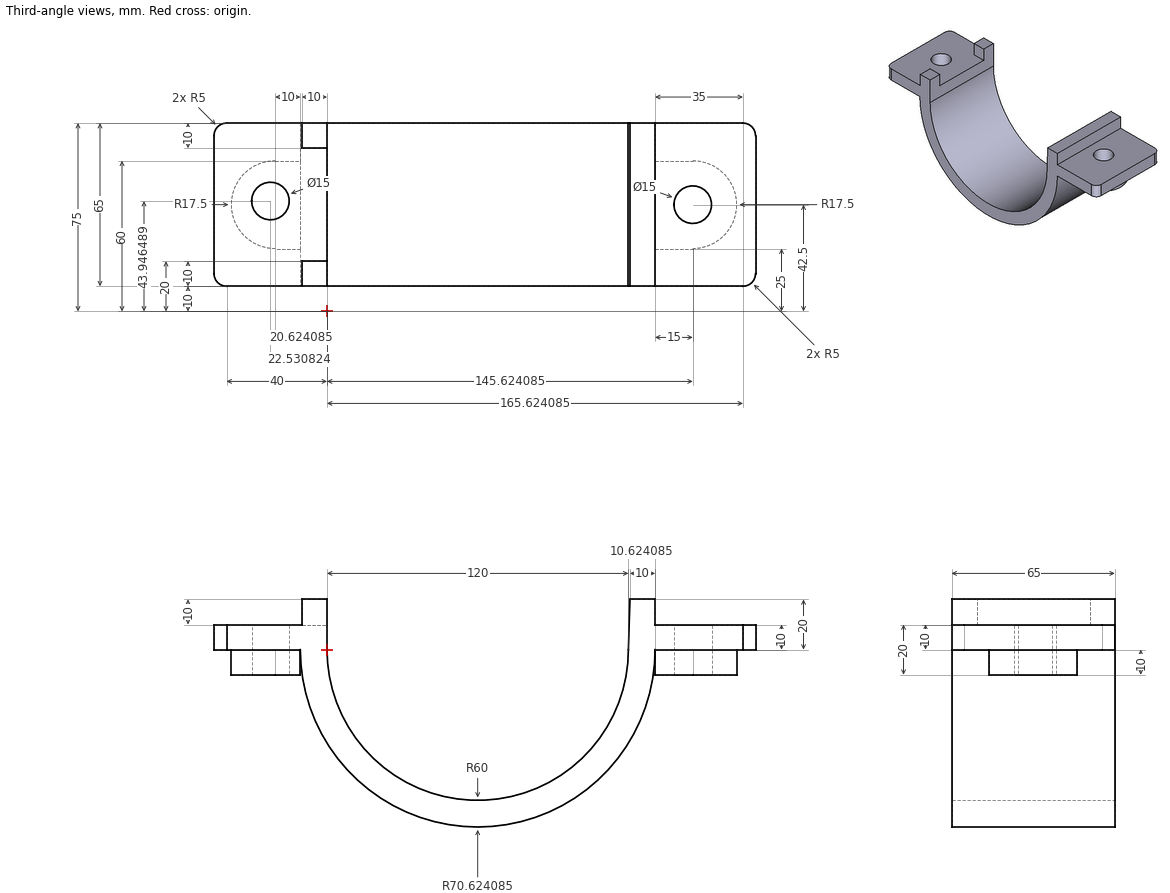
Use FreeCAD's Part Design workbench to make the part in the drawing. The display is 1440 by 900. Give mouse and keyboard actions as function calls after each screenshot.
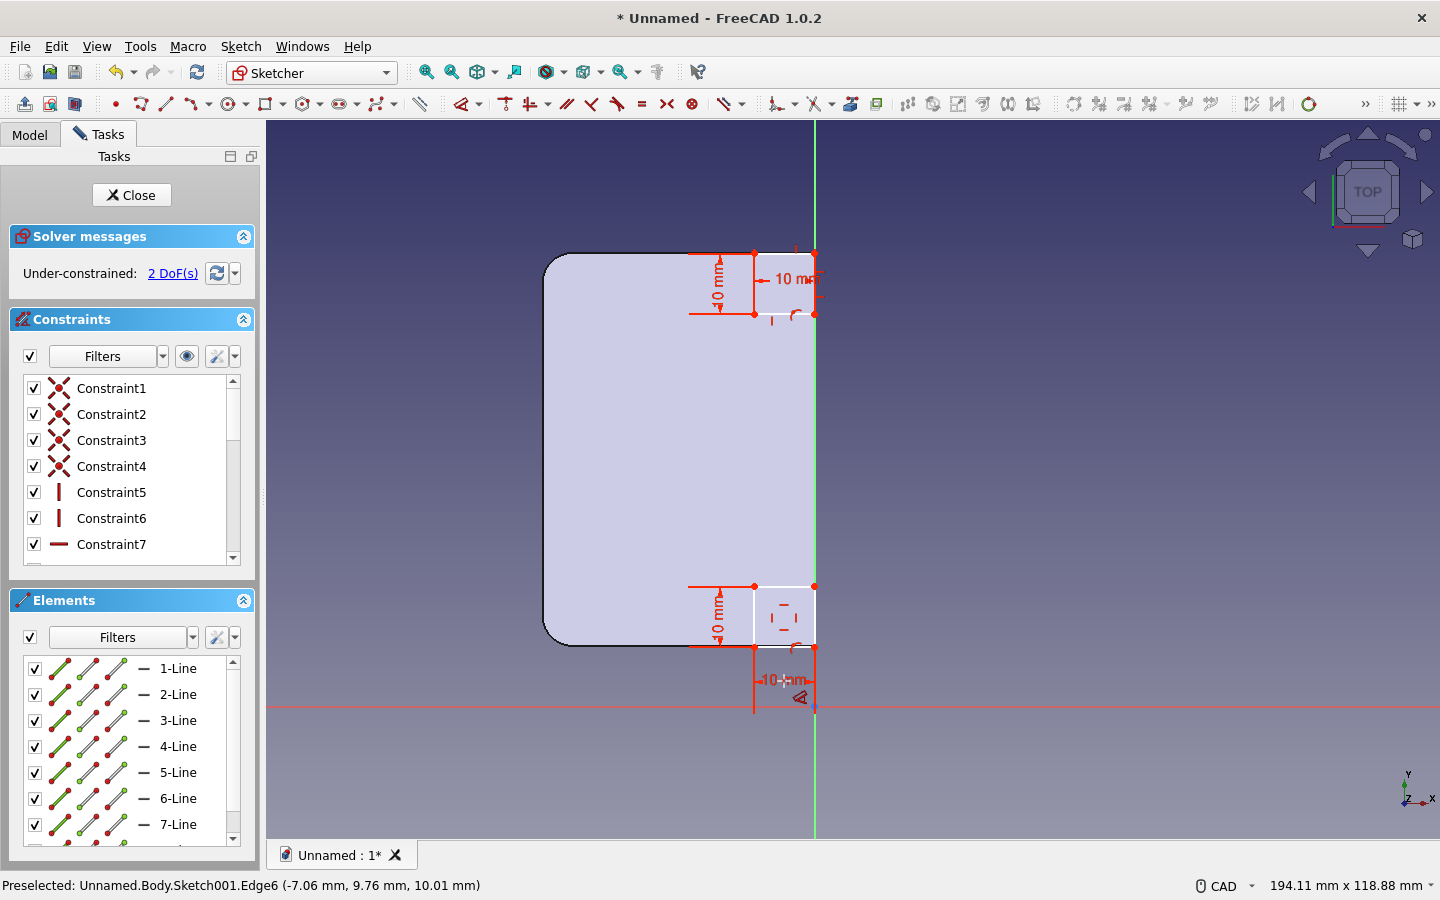
click(754, 254)
click(849, 480)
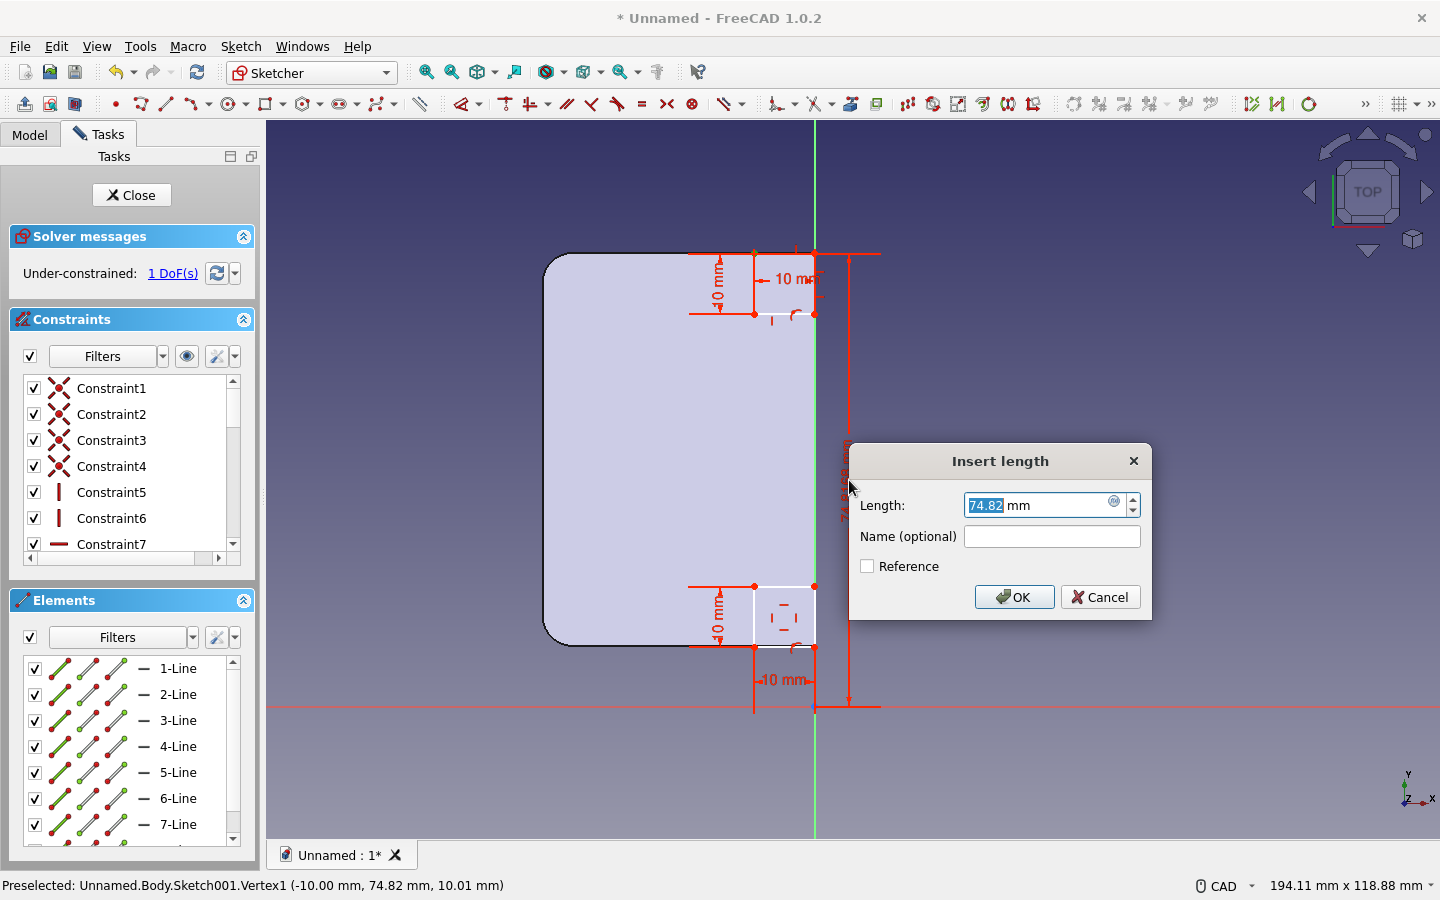
text(75)
key(Return)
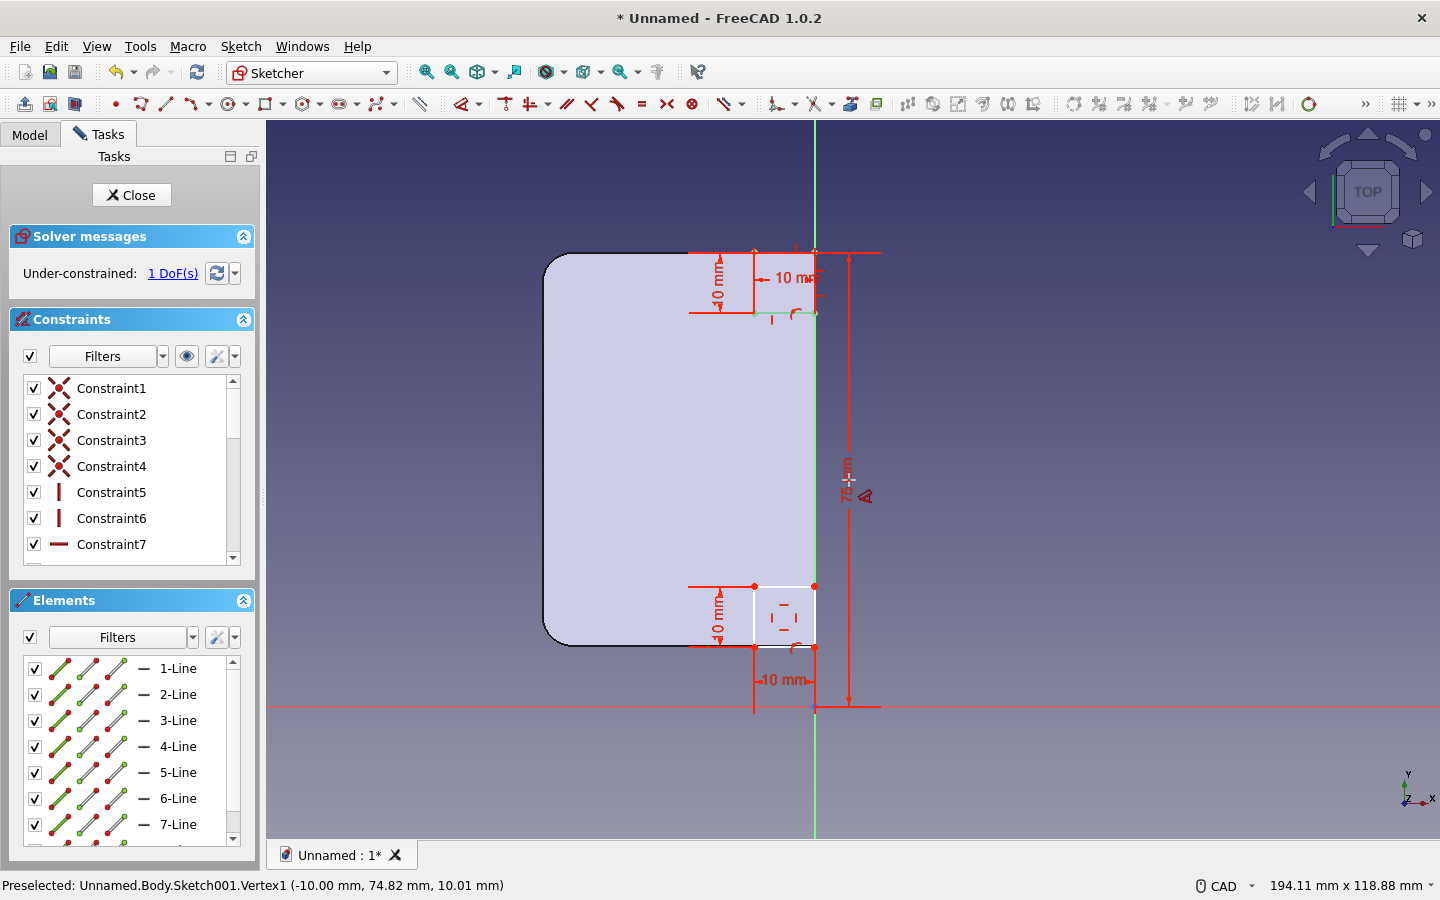
click(754, 587)
click(849, 647)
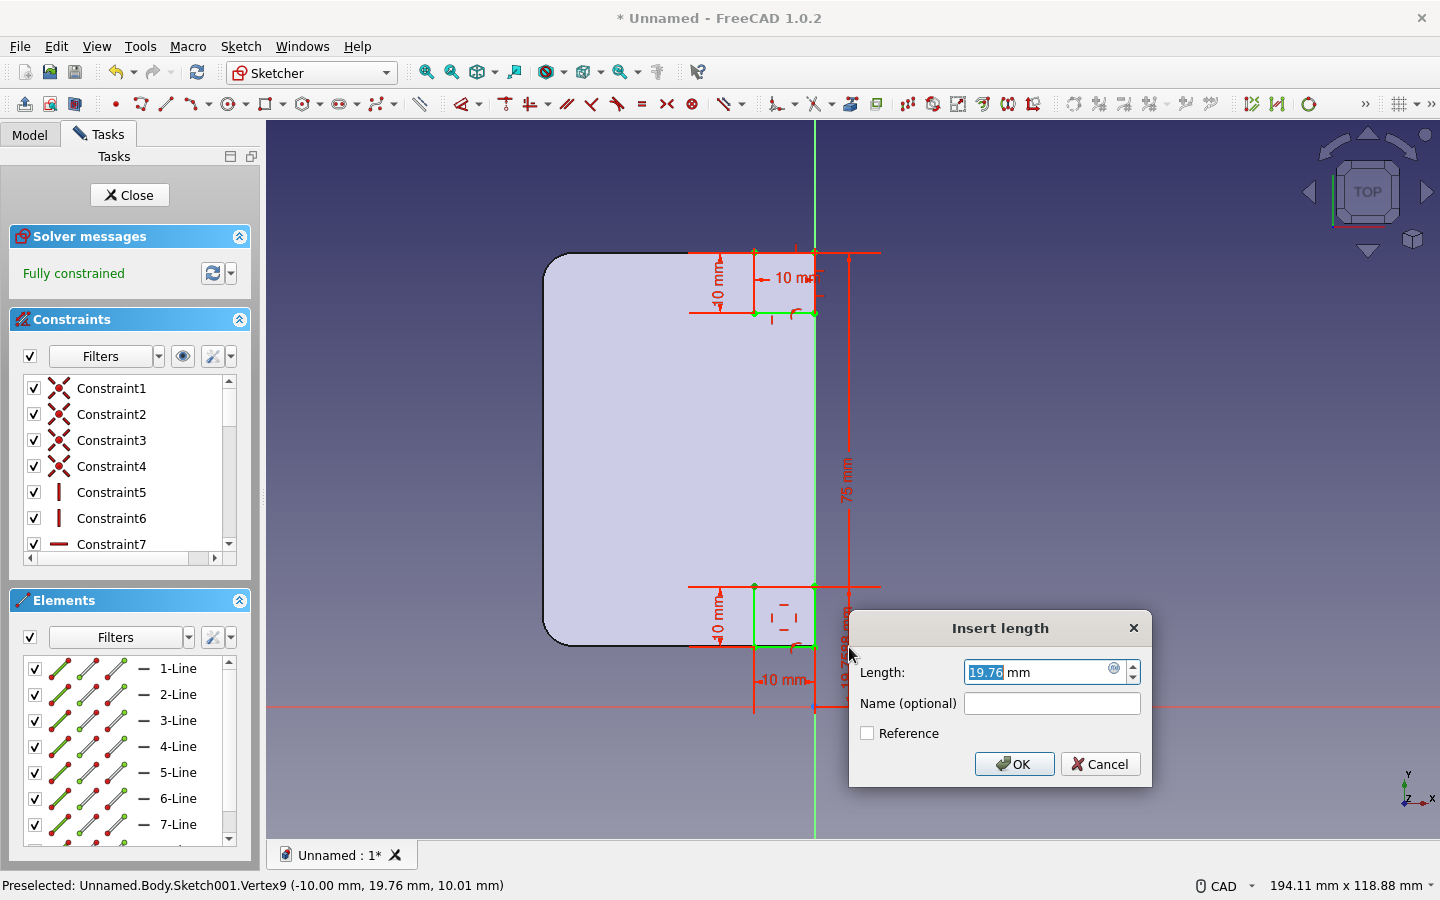
text(20)
key(Return)
key(Escape)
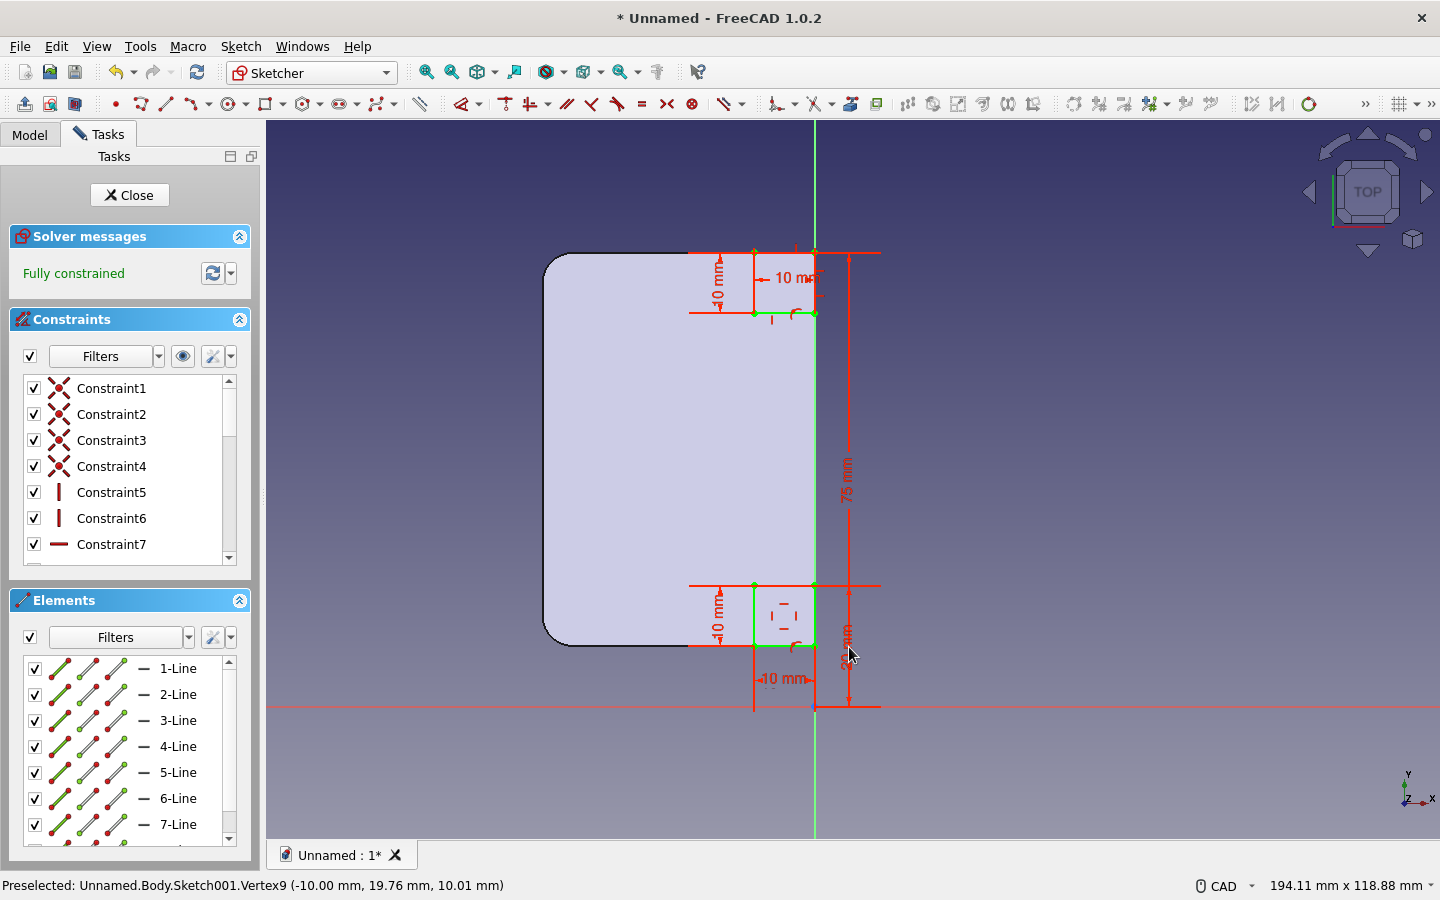
click(130, 195)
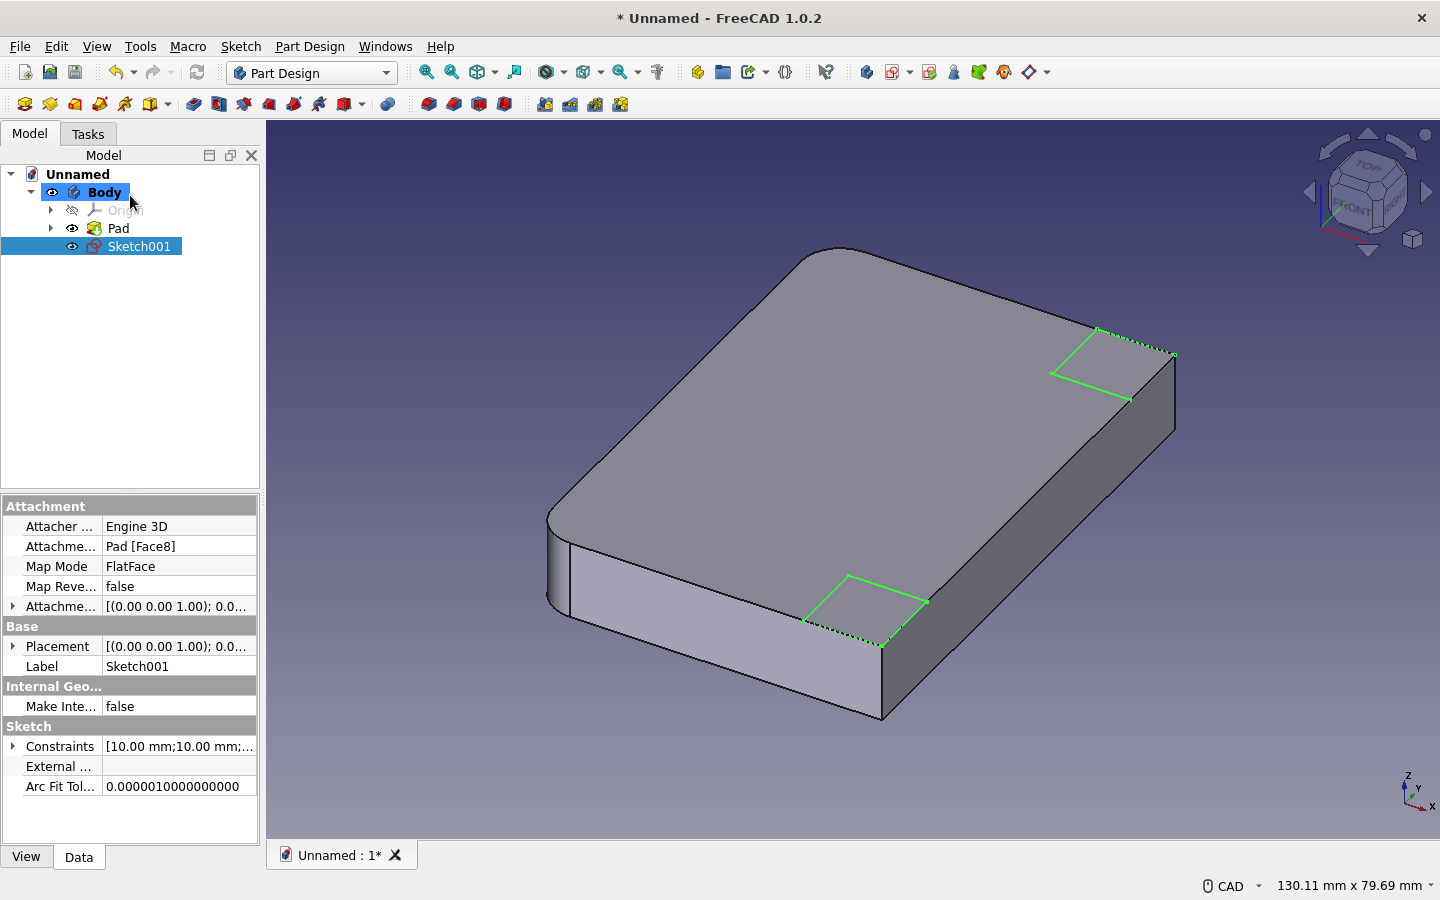
click(25, 104)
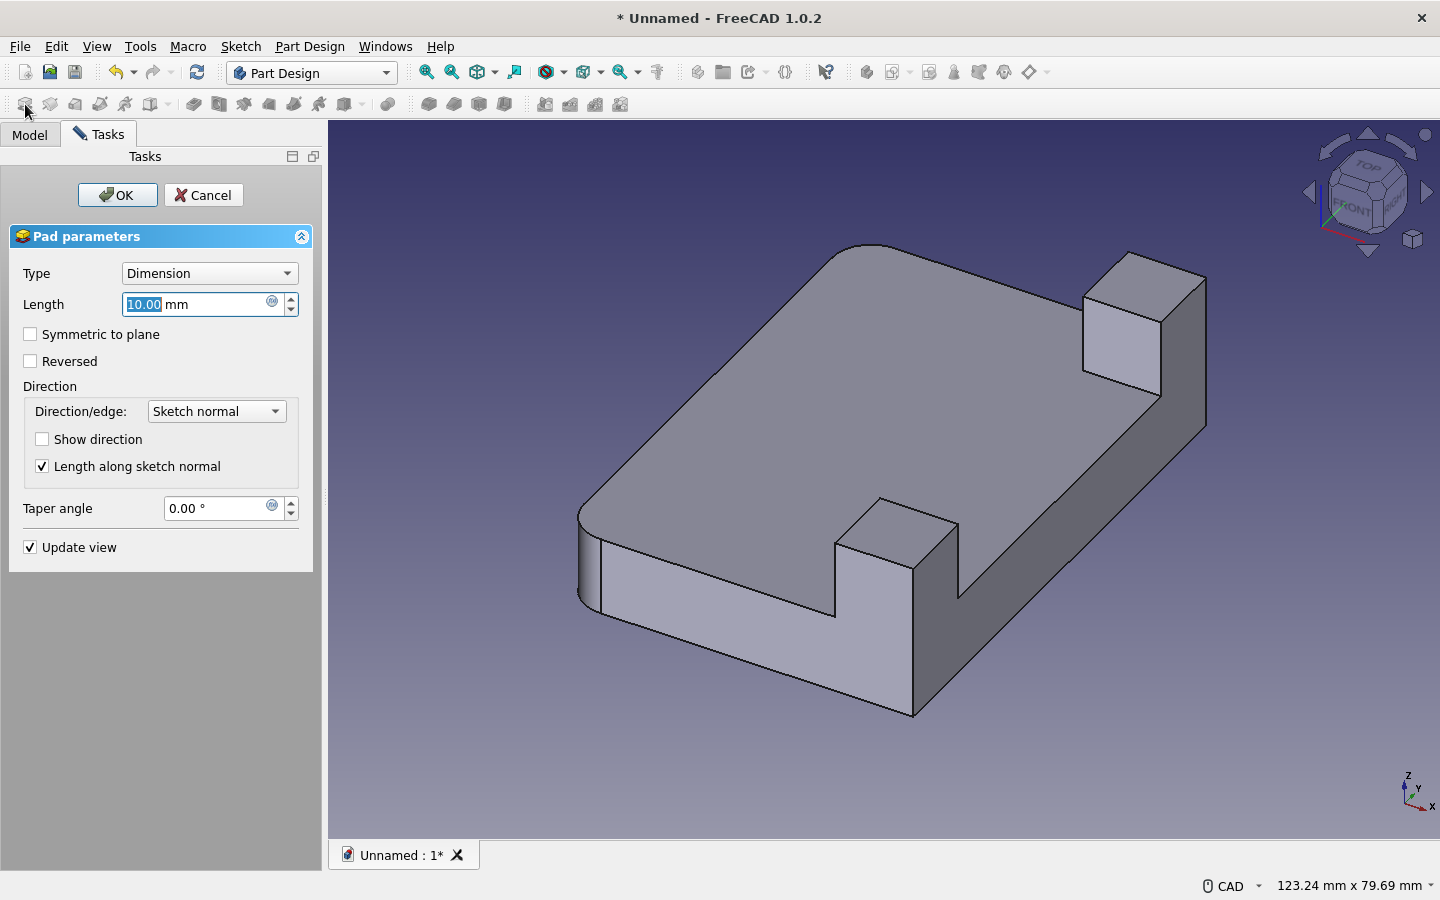
text(10)
key(Tab)